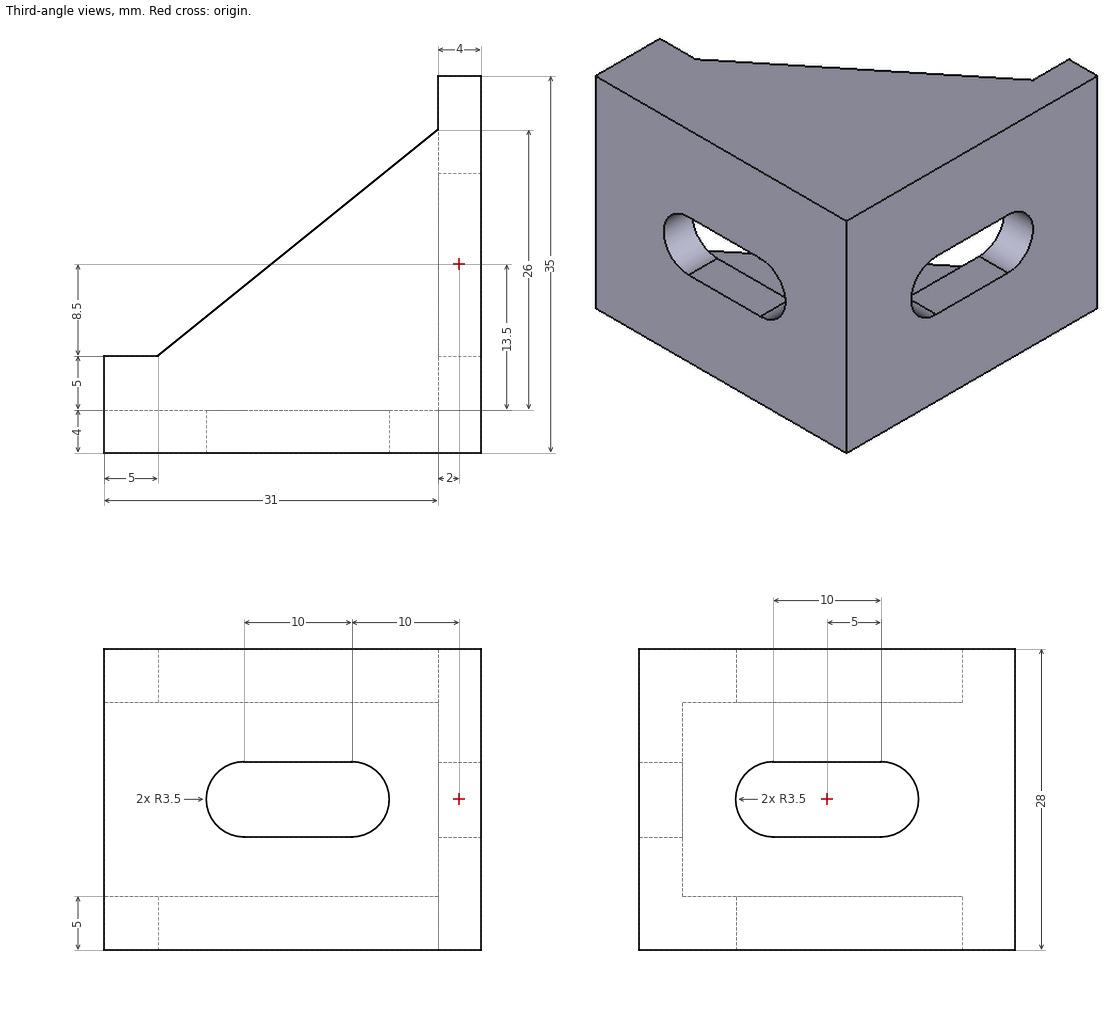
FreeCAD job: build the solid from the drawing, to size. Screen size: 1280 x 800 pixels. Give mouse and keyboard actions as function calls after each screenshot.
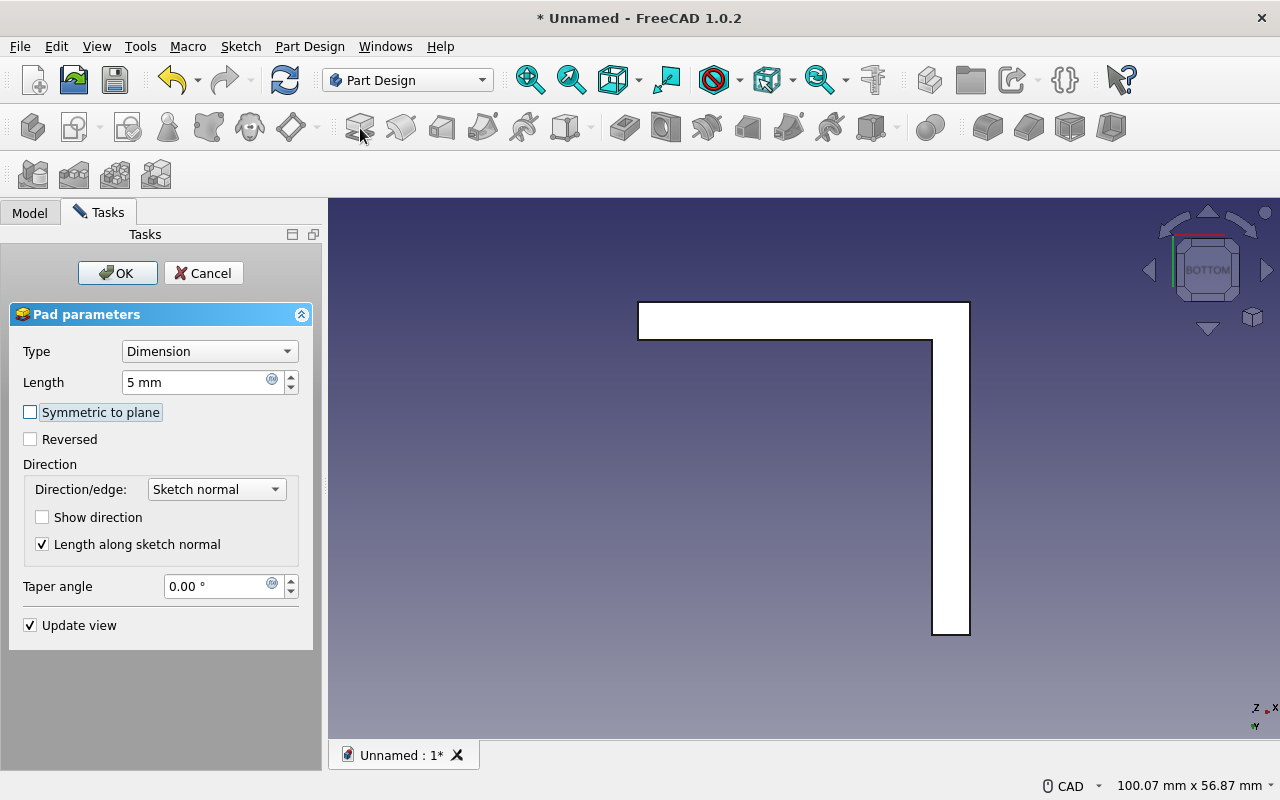
click(31, 439)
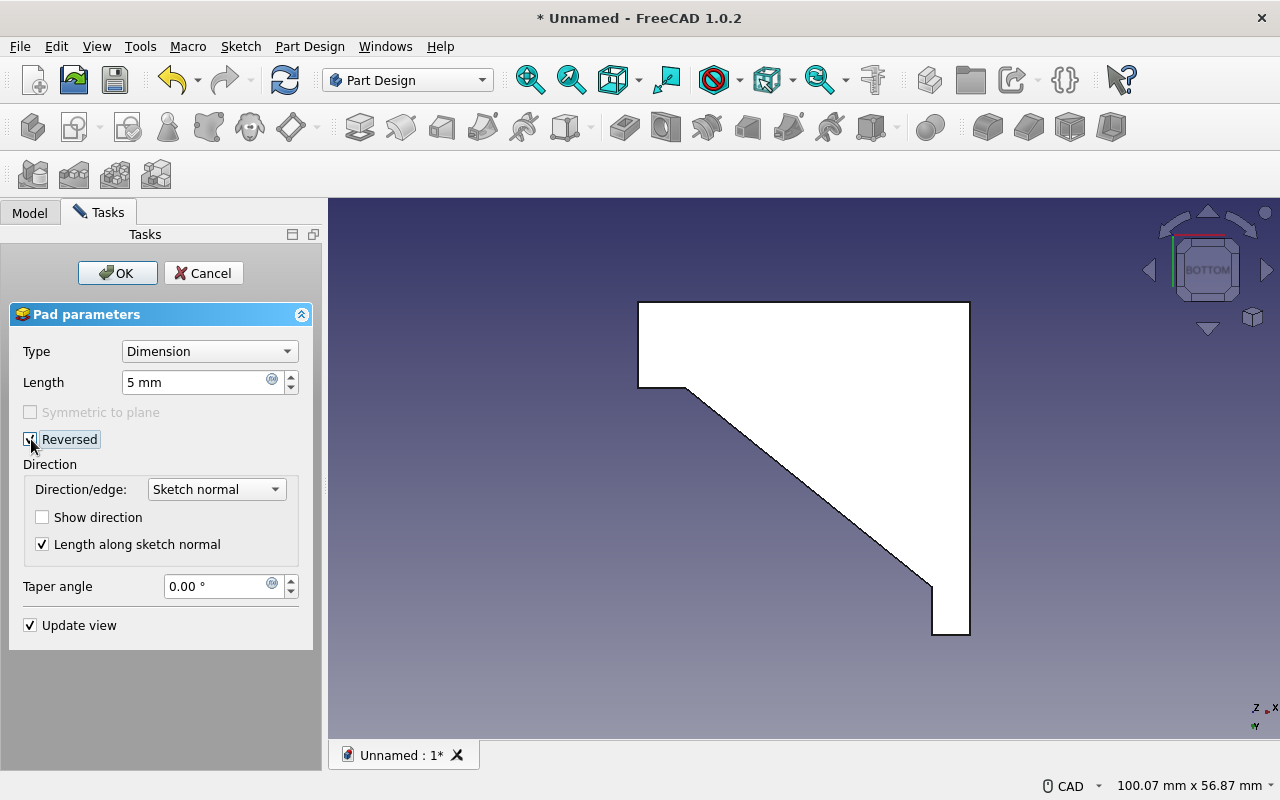
click(118, 273)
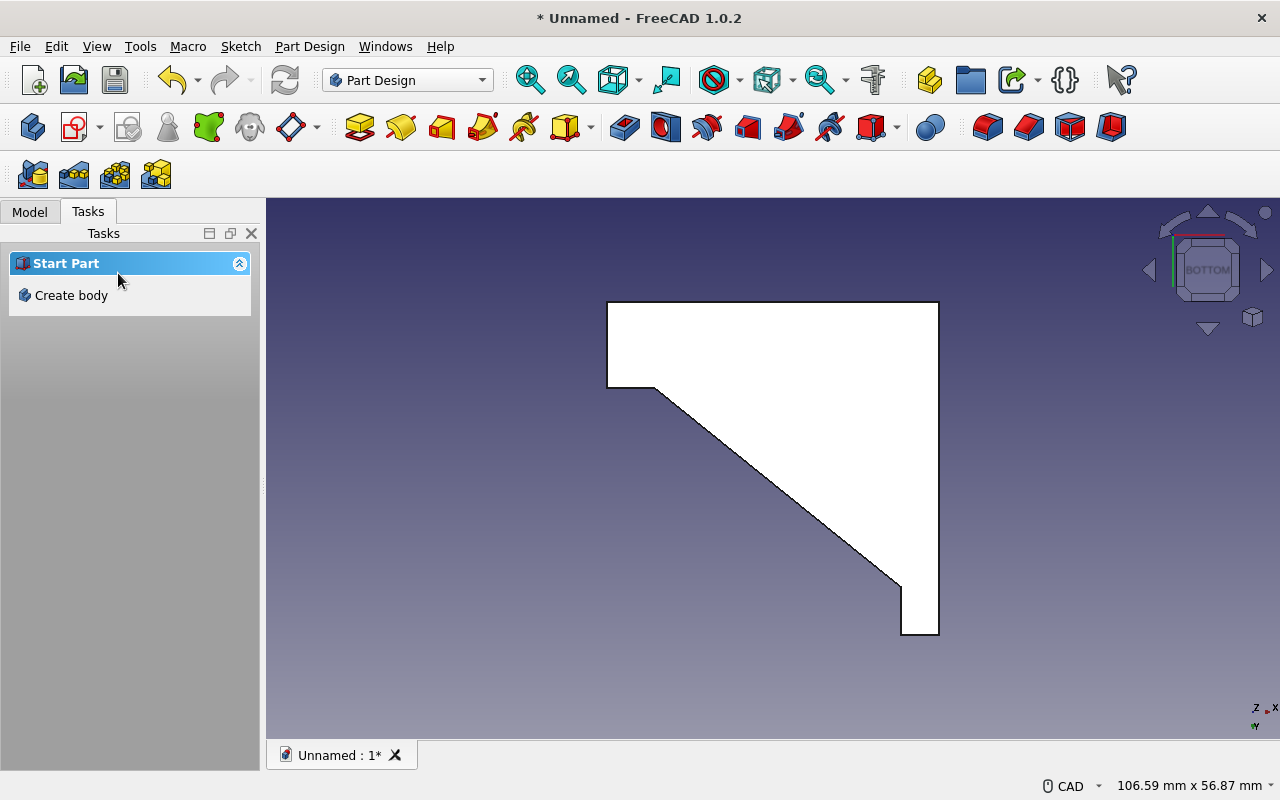
click(30, 212)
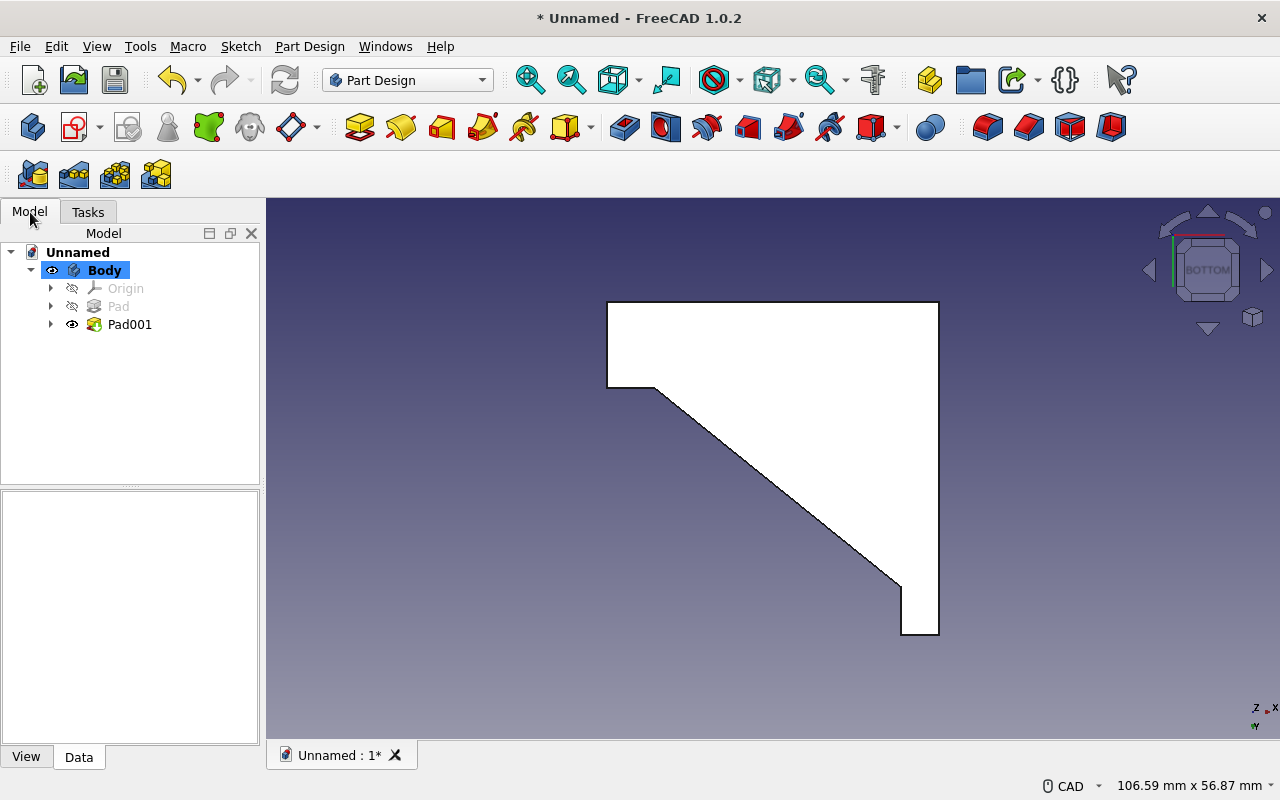
click(117, 324)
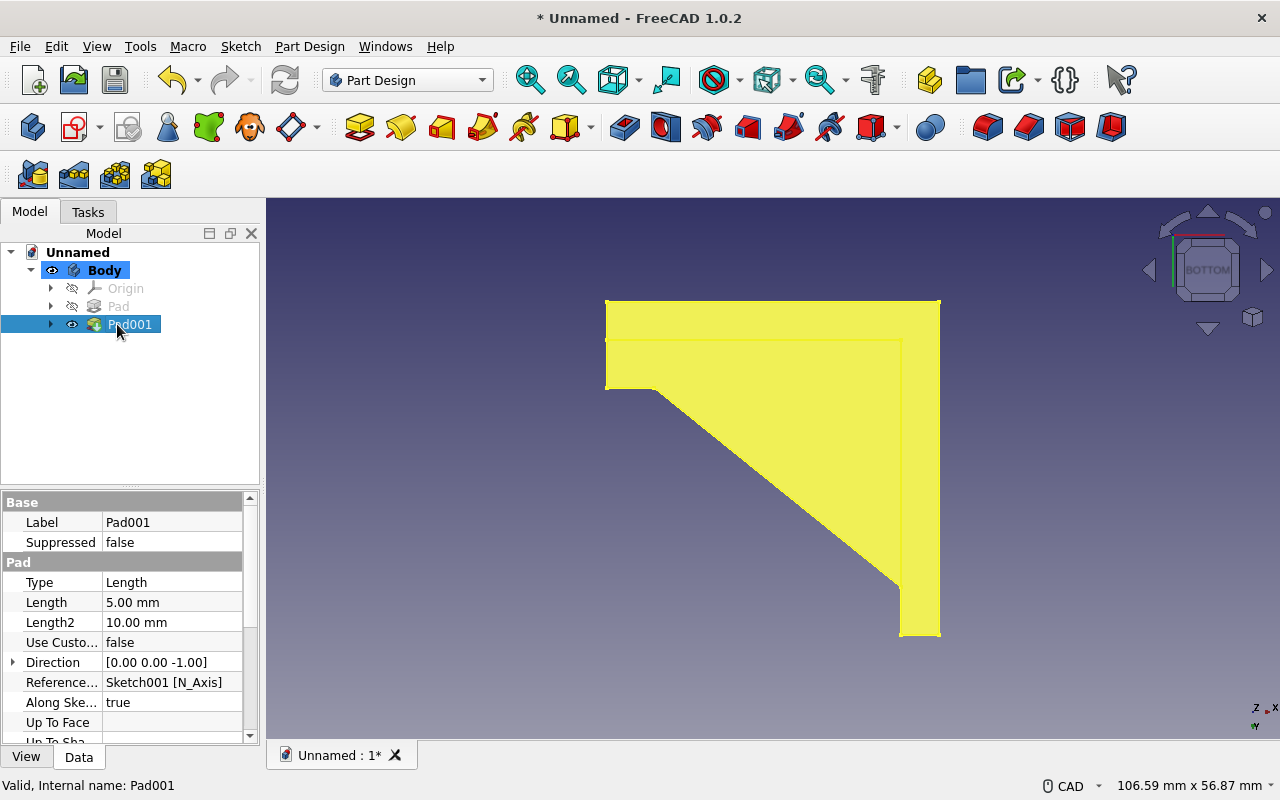
click(33, 174)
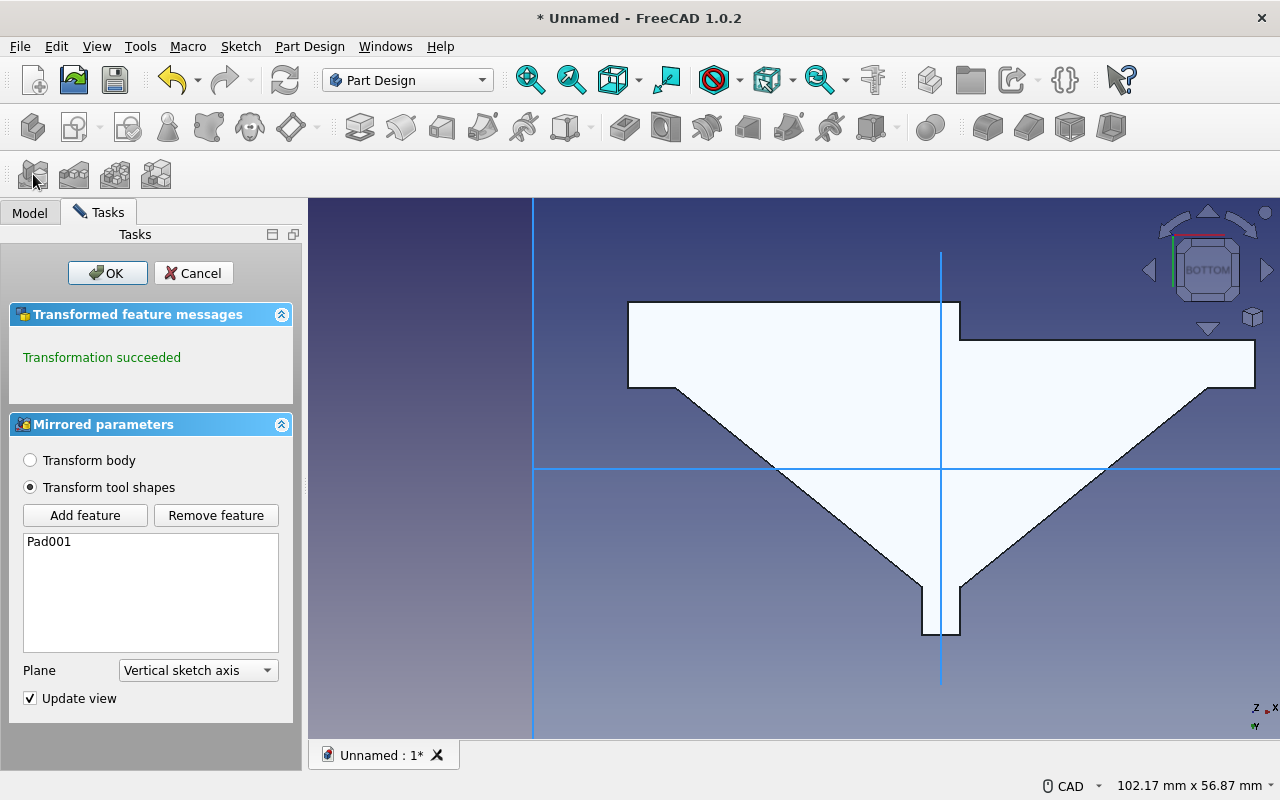
click(199, 670)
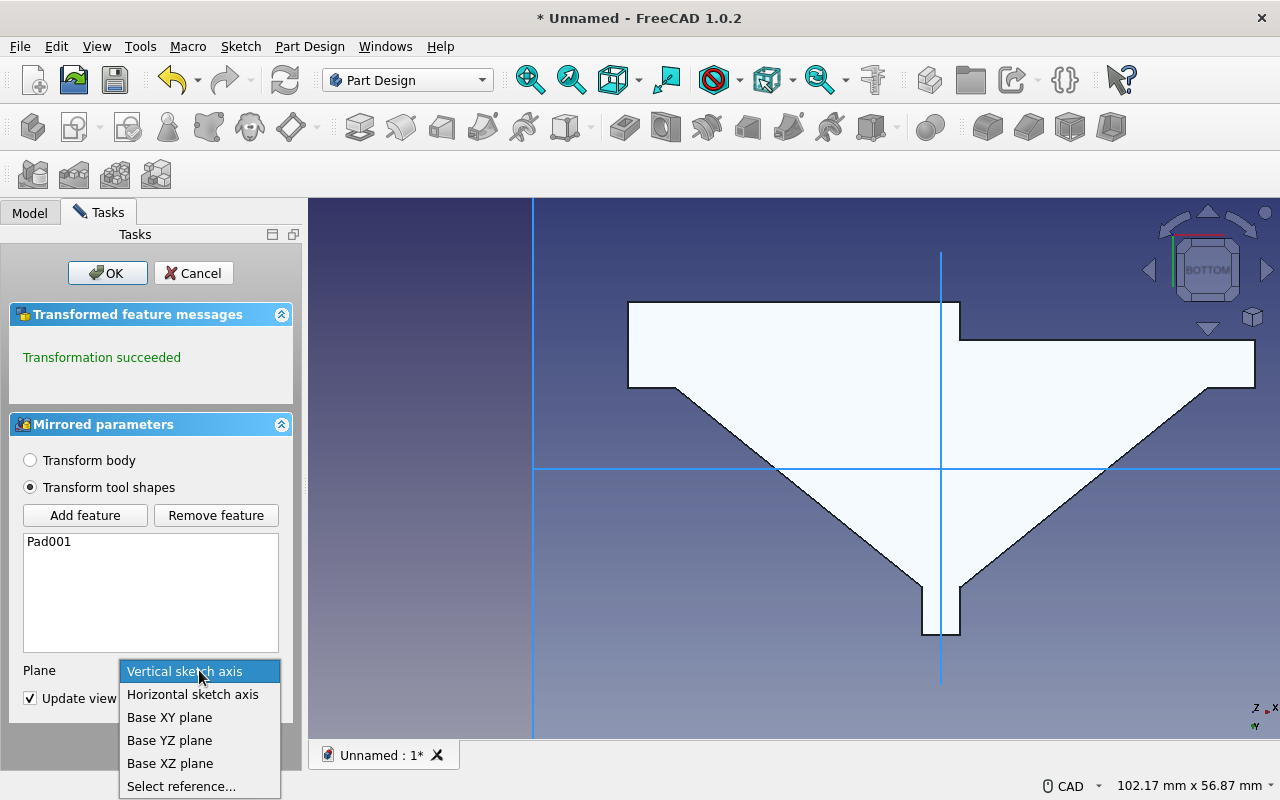
click(198, 718)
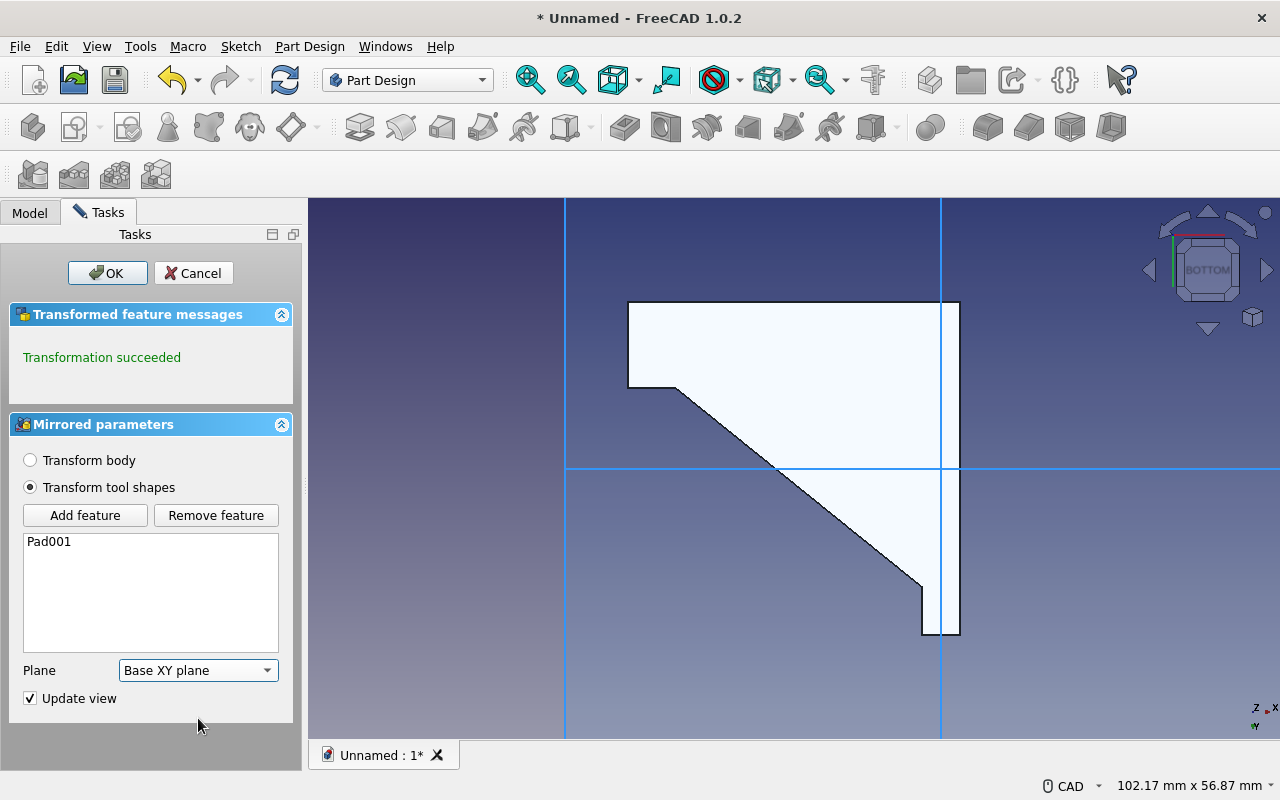
click(108, 273)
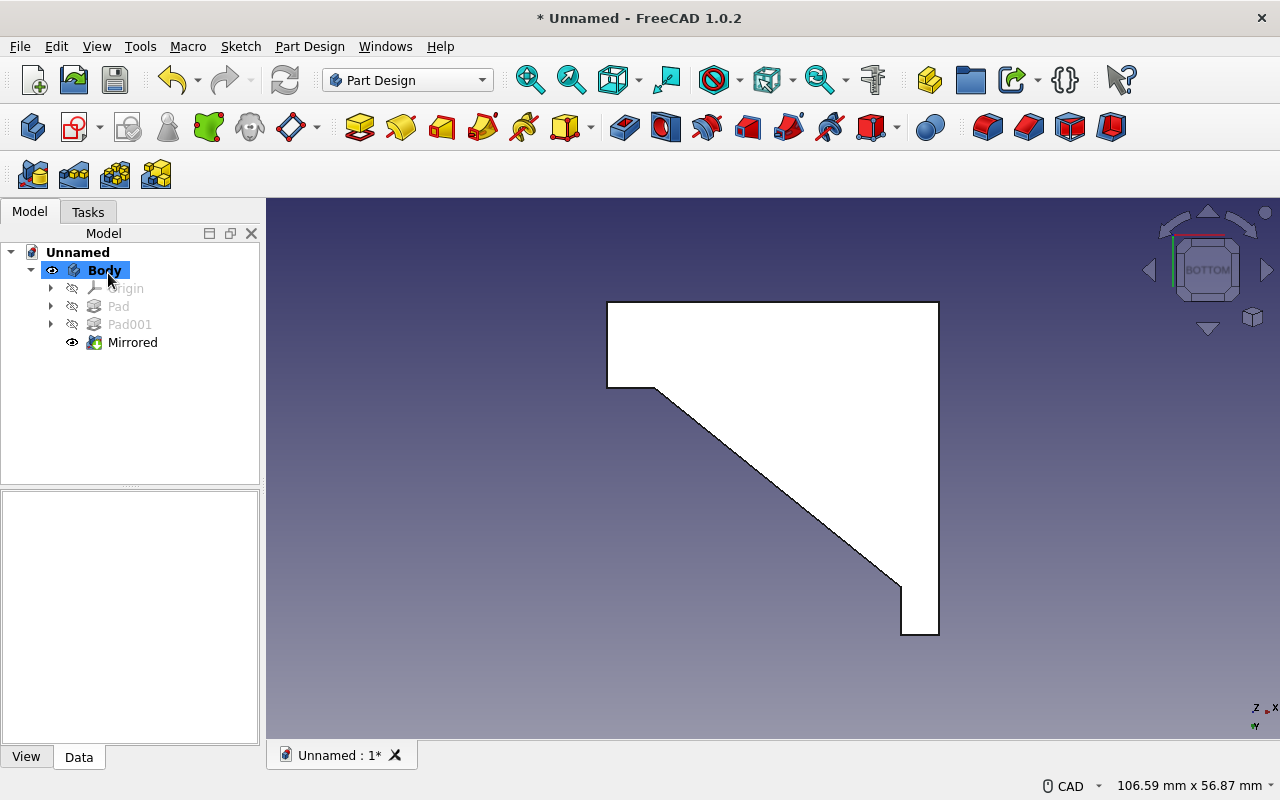
key(6)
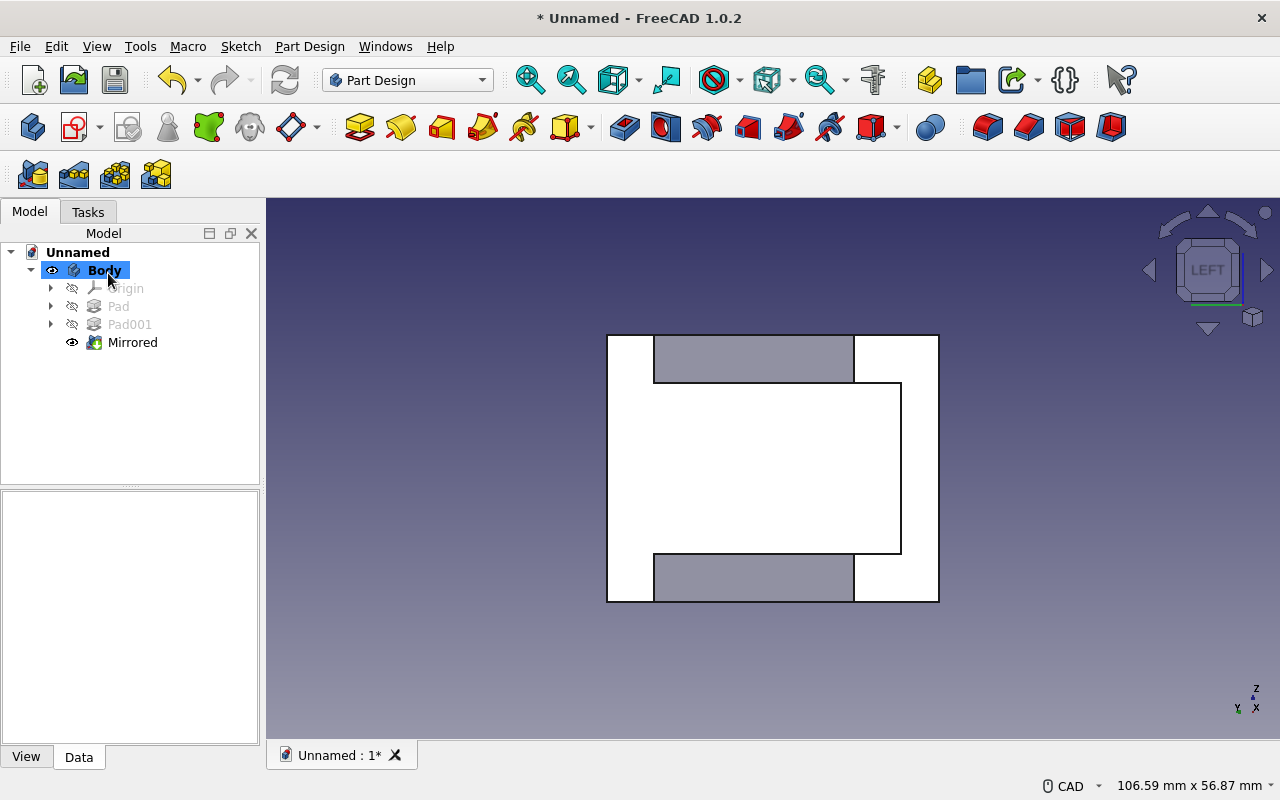
click(712, 467)